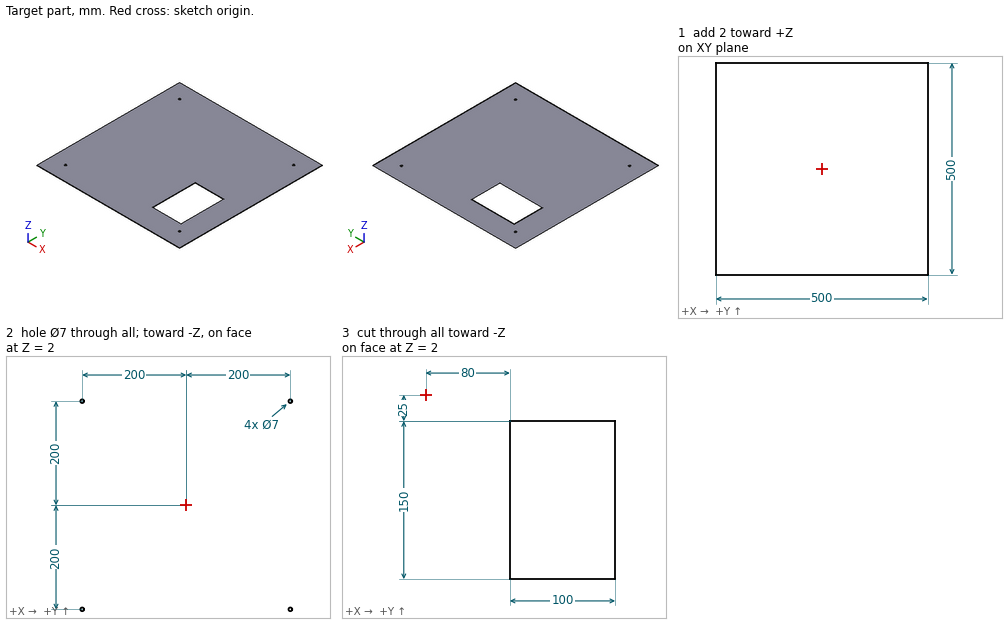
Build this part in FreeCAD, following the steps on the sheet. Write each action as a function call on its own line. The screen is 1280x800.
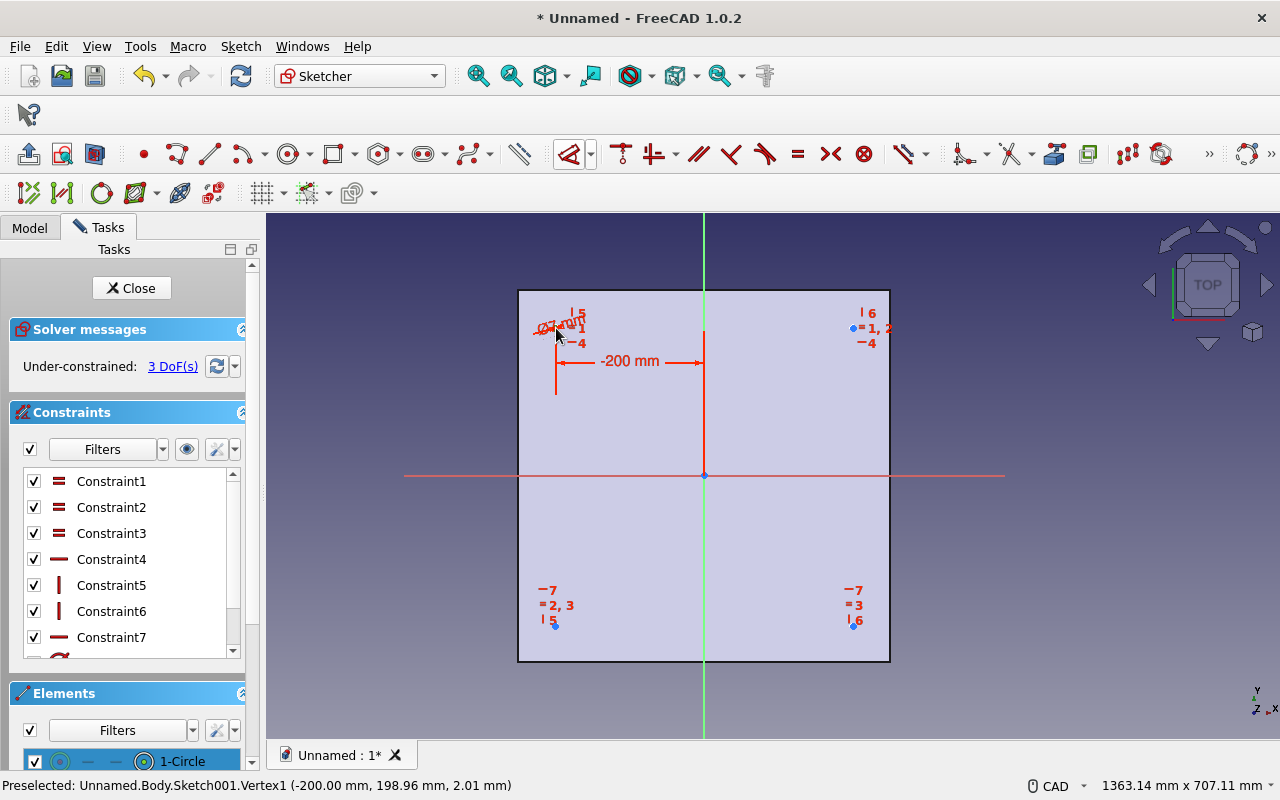
click(590, 154)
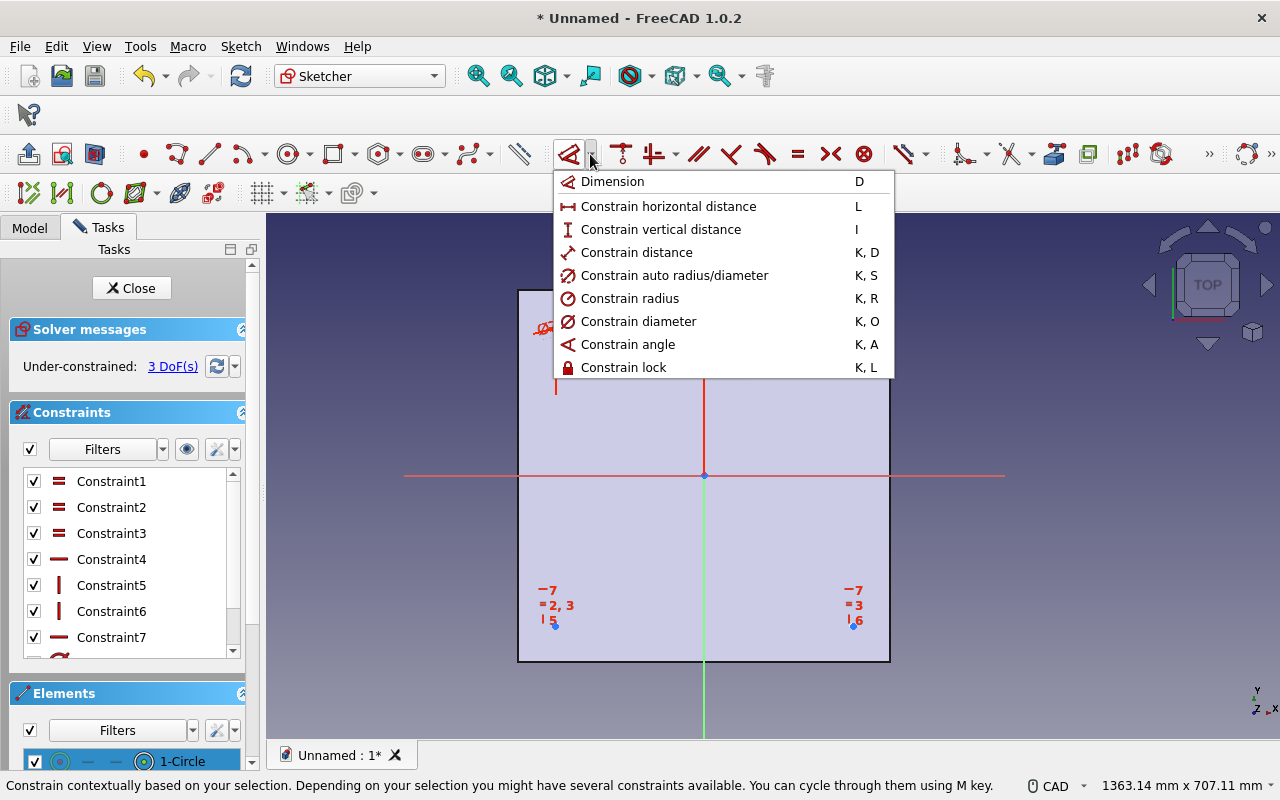
click(724, 230)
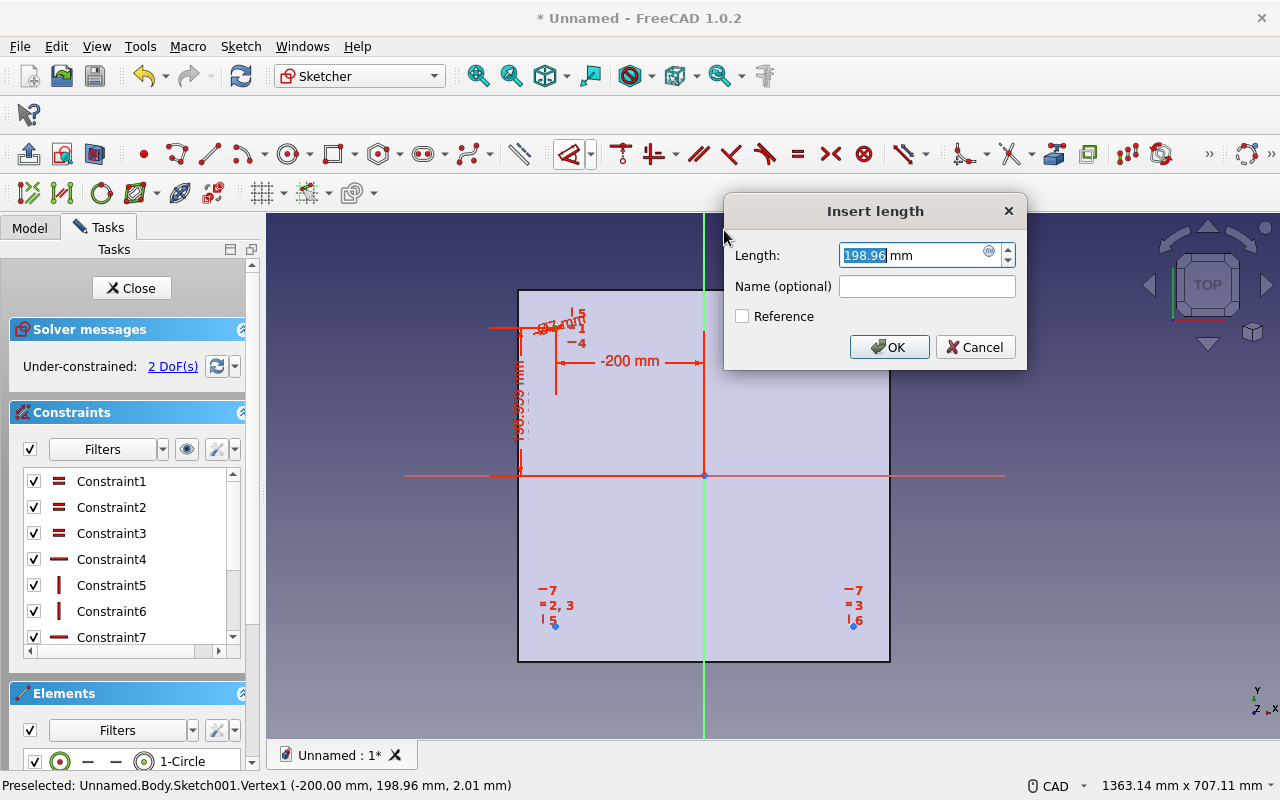
text(200)
key(Return)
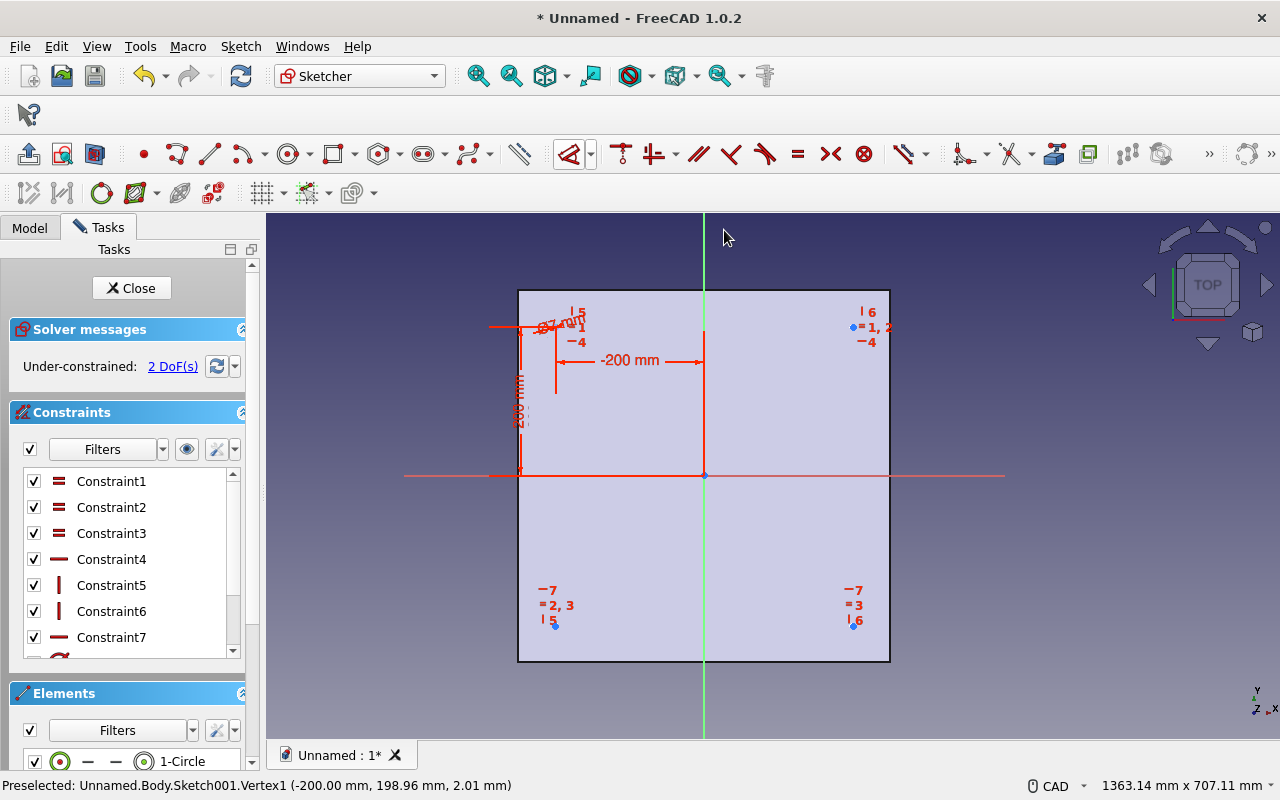
click(853, 327)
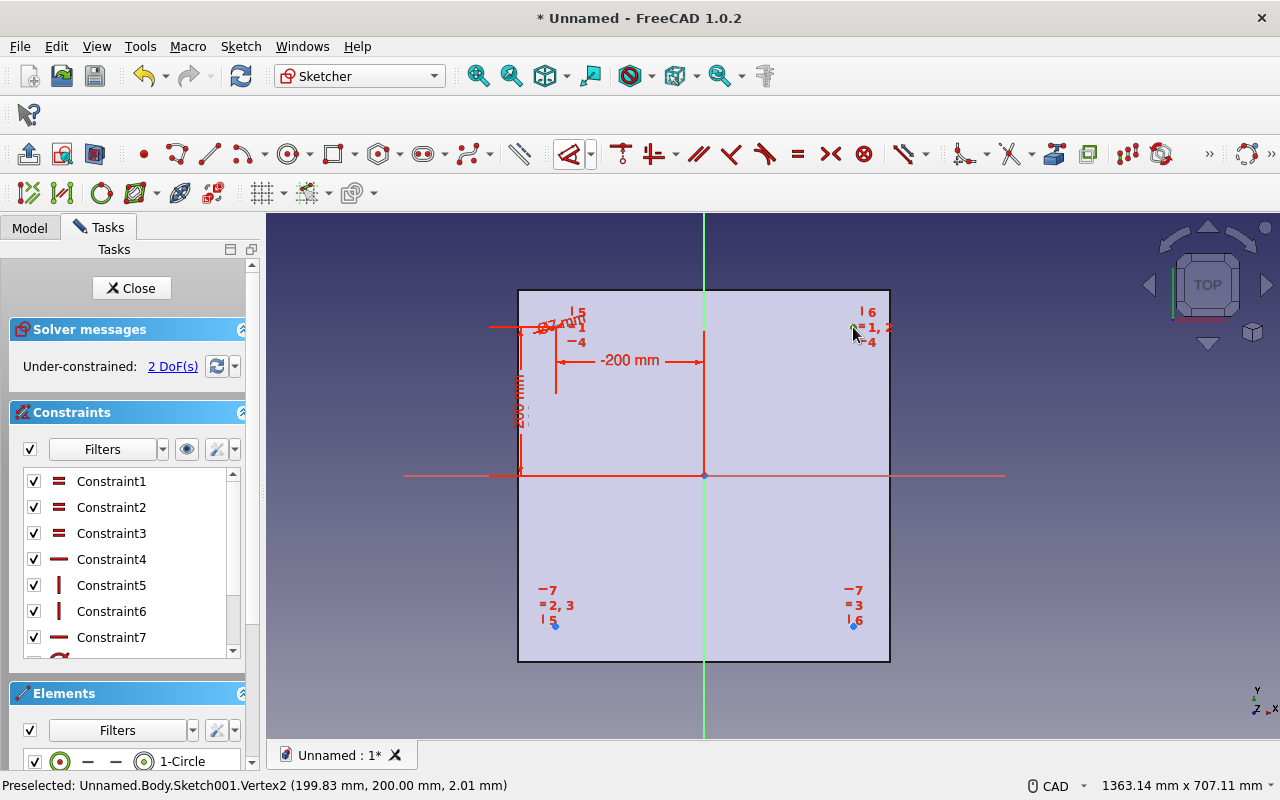
key(l)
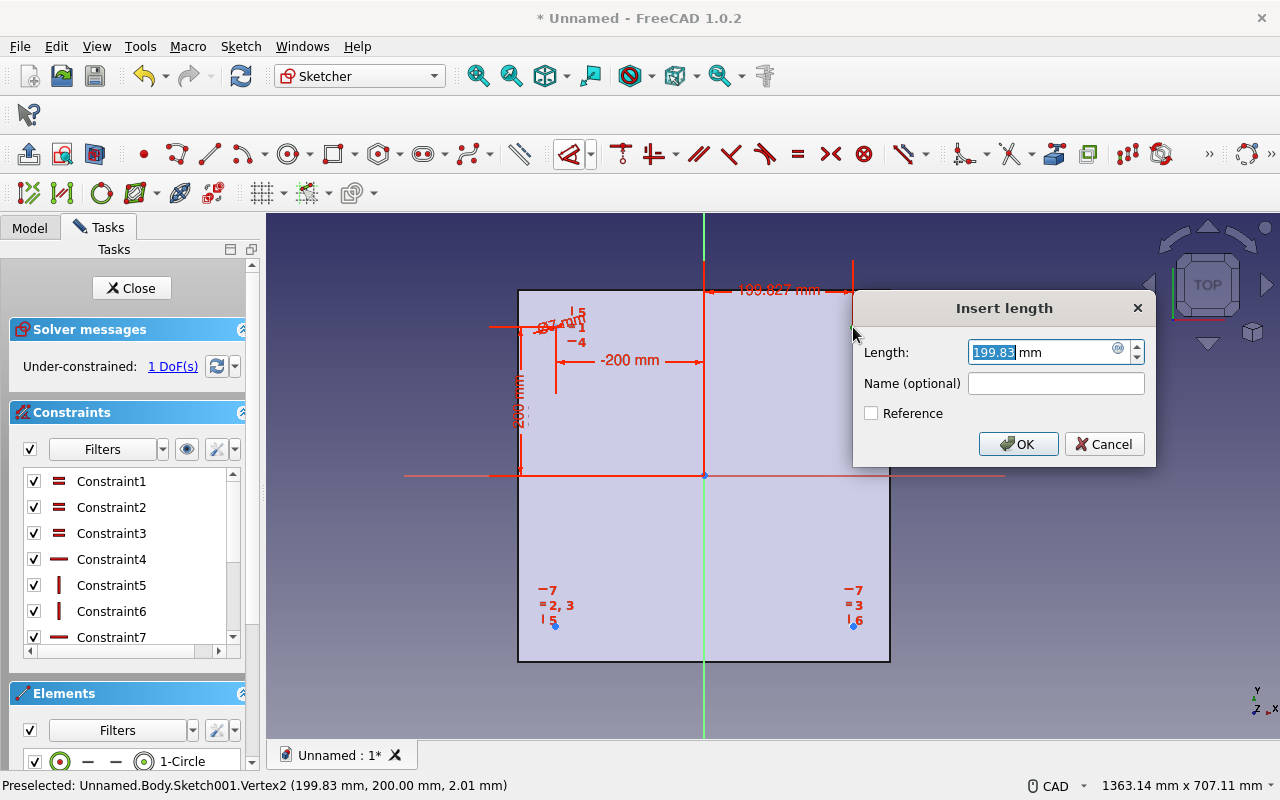
text(200)
key(Return)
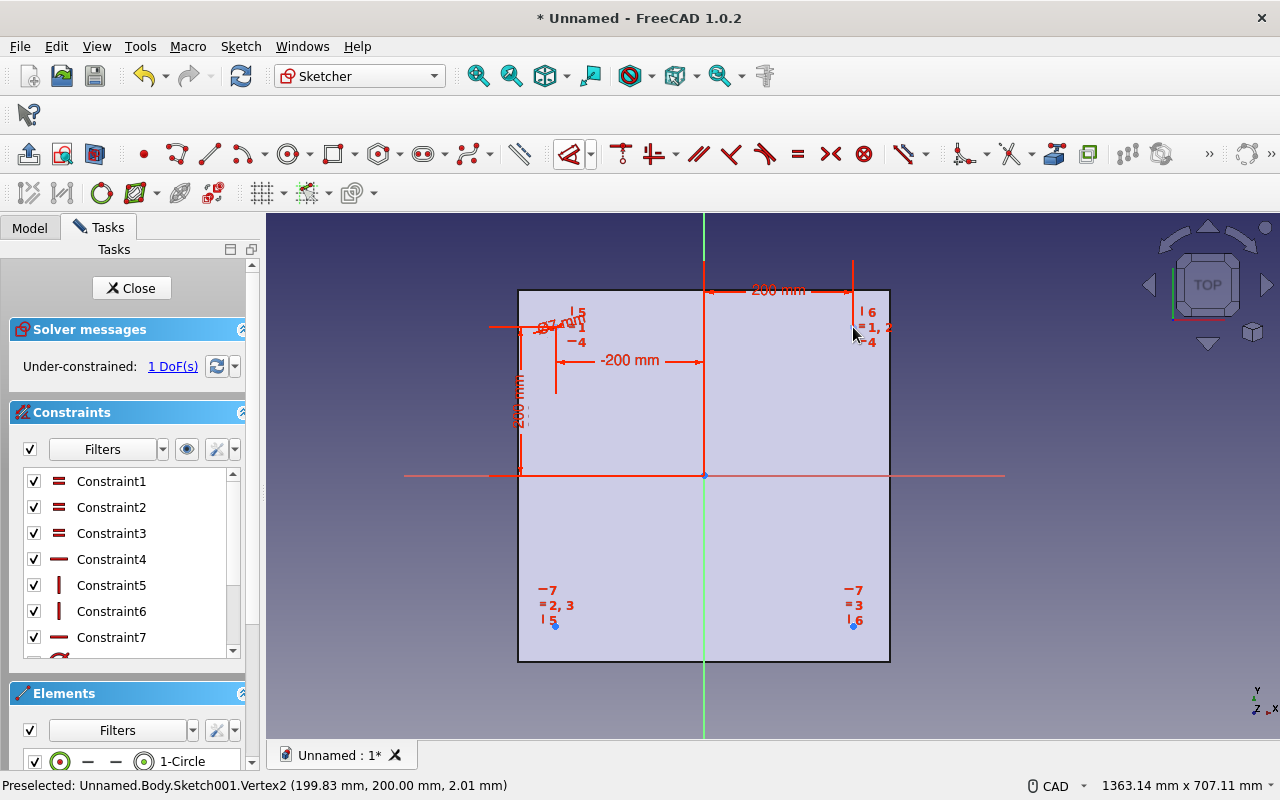
click(556, 626)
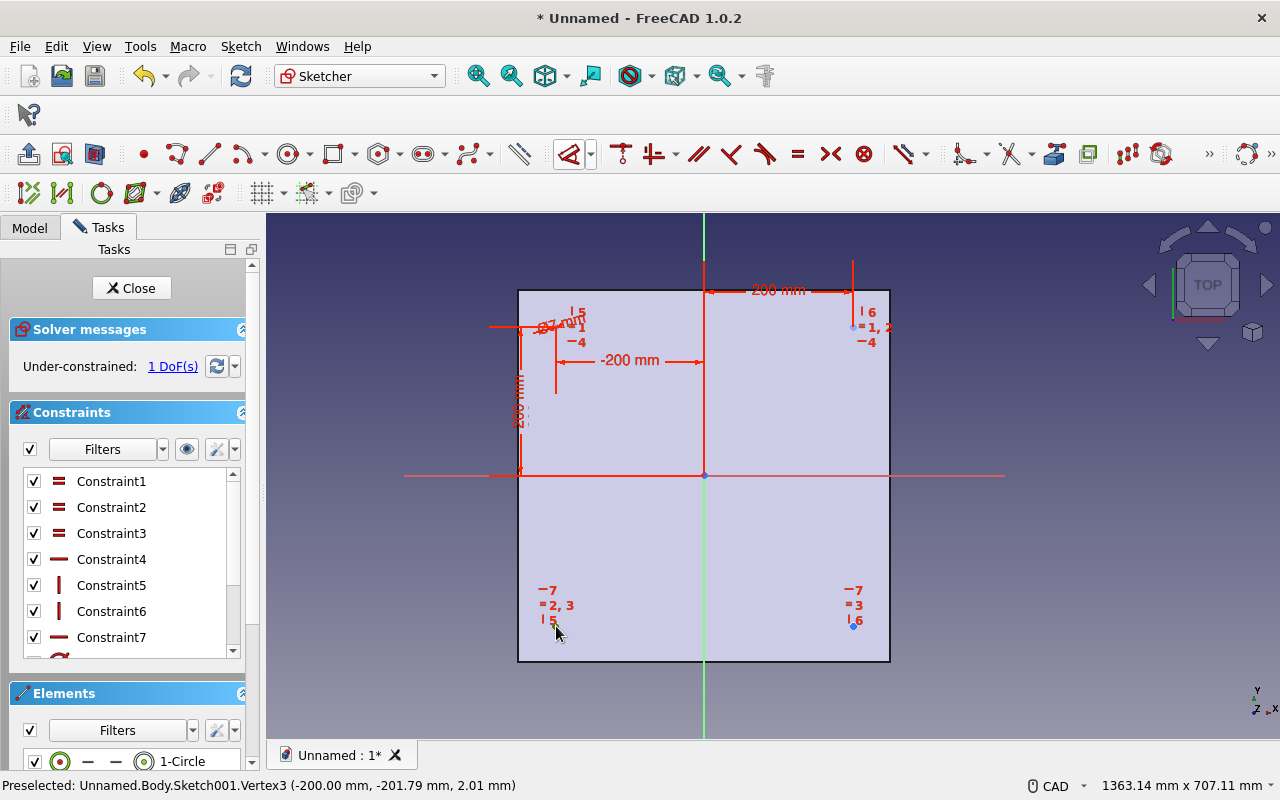
key(i)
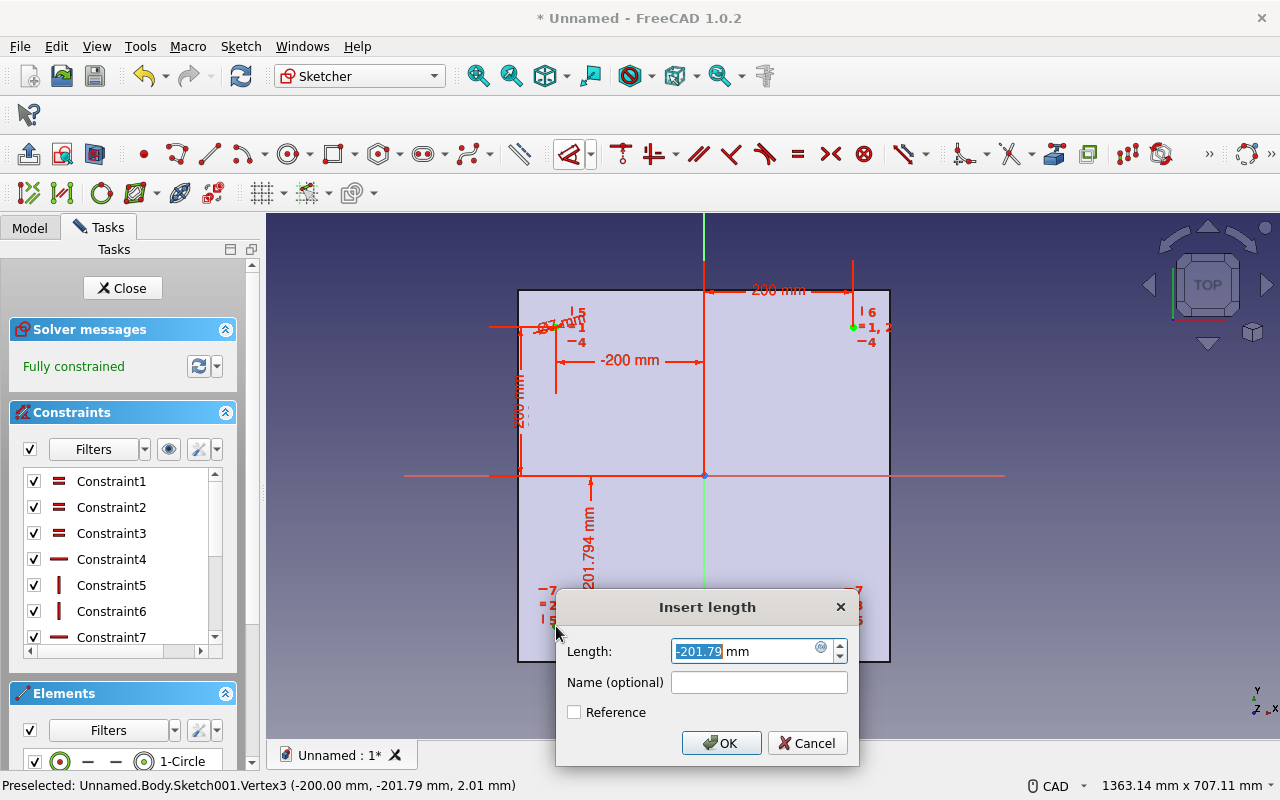
text(-200)
key(Return)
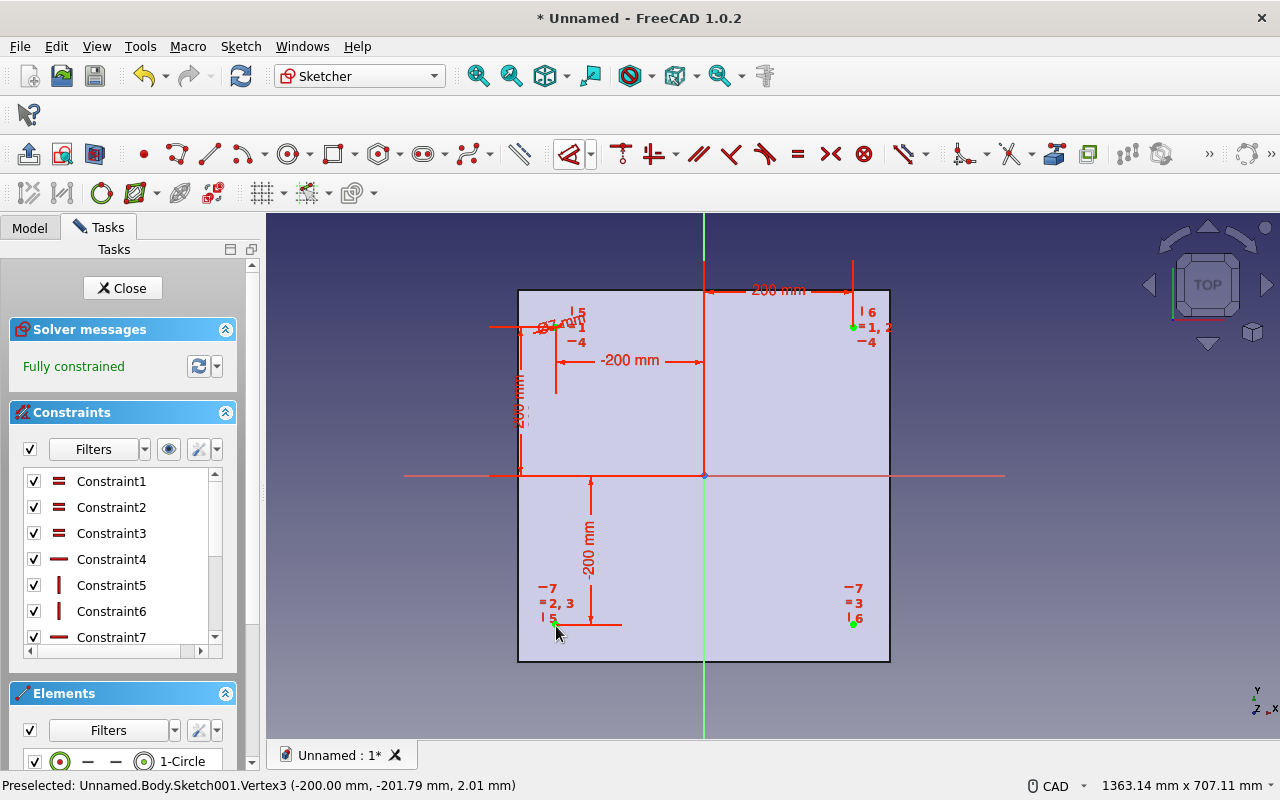
click(123, 288)